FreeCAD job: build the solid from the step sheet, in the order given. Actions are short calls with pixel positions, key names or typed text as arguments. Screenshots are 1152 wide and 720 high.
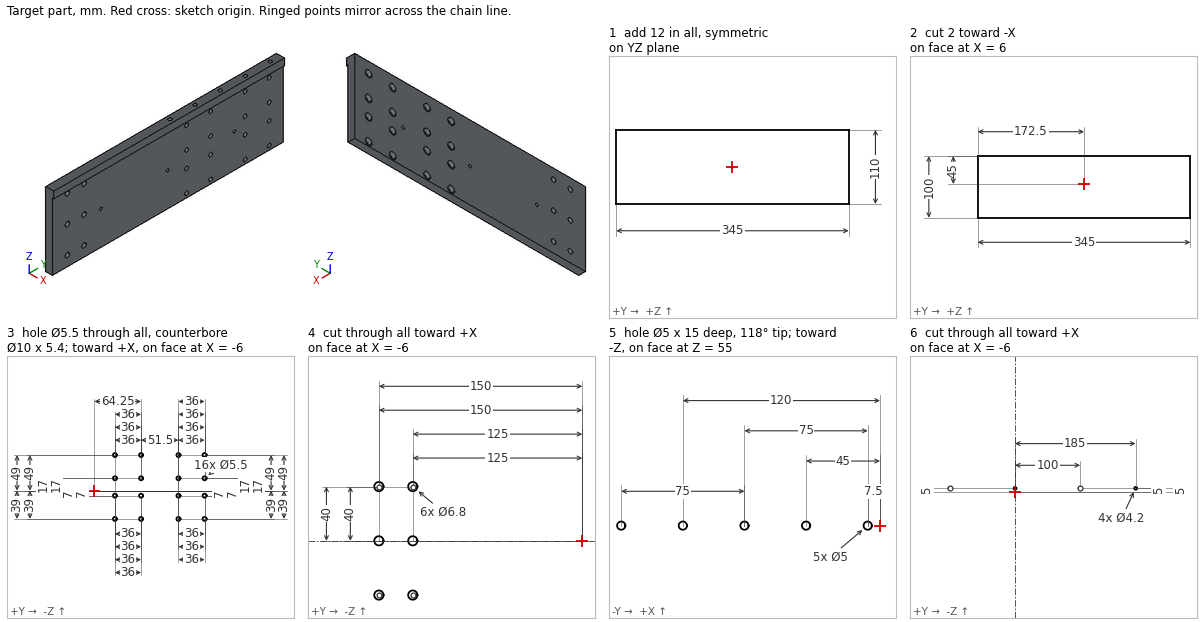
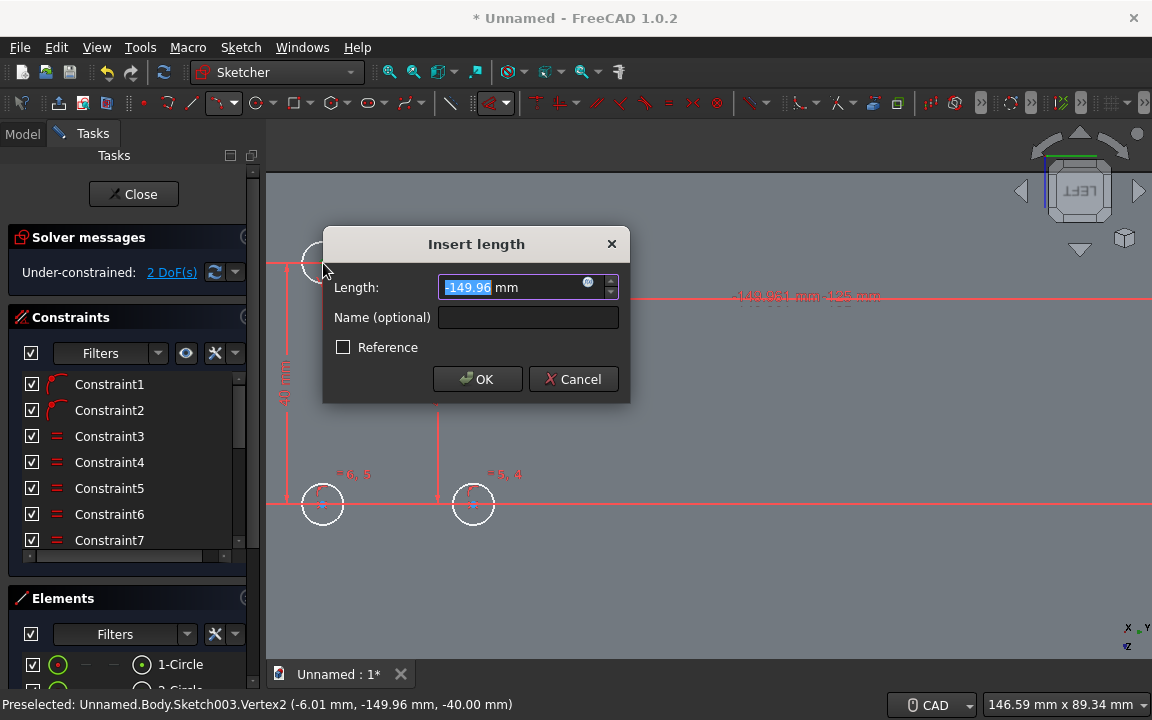
text(-150)
key(Return)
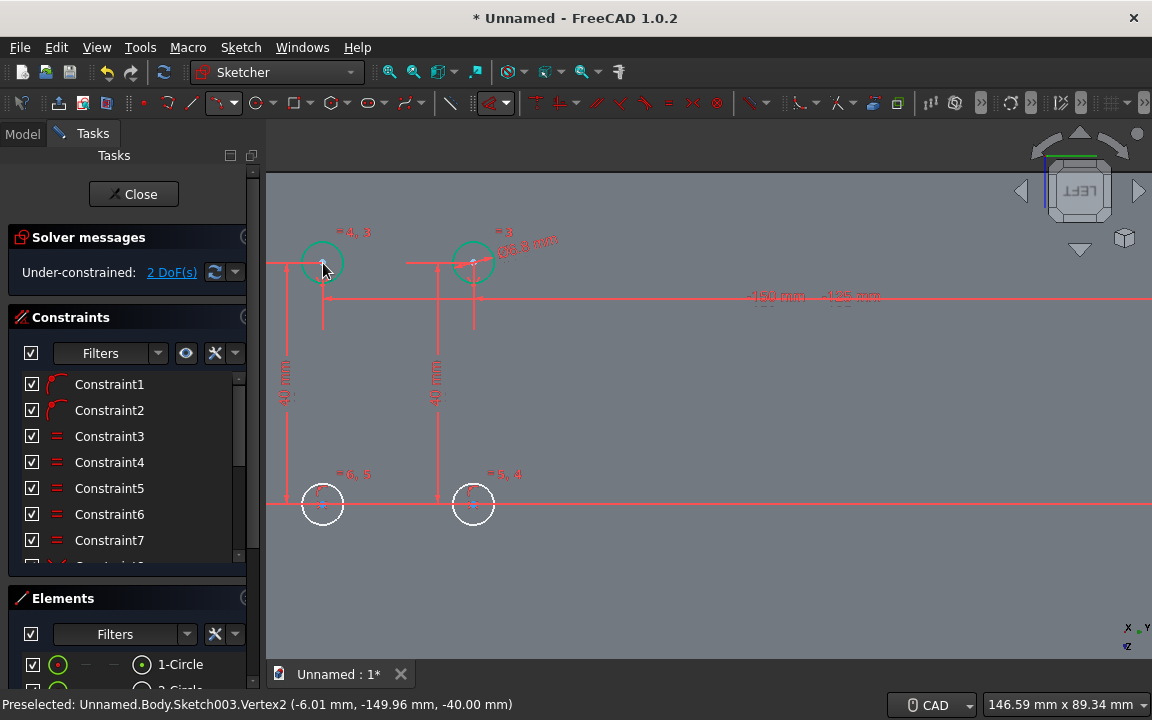
click(473, 504)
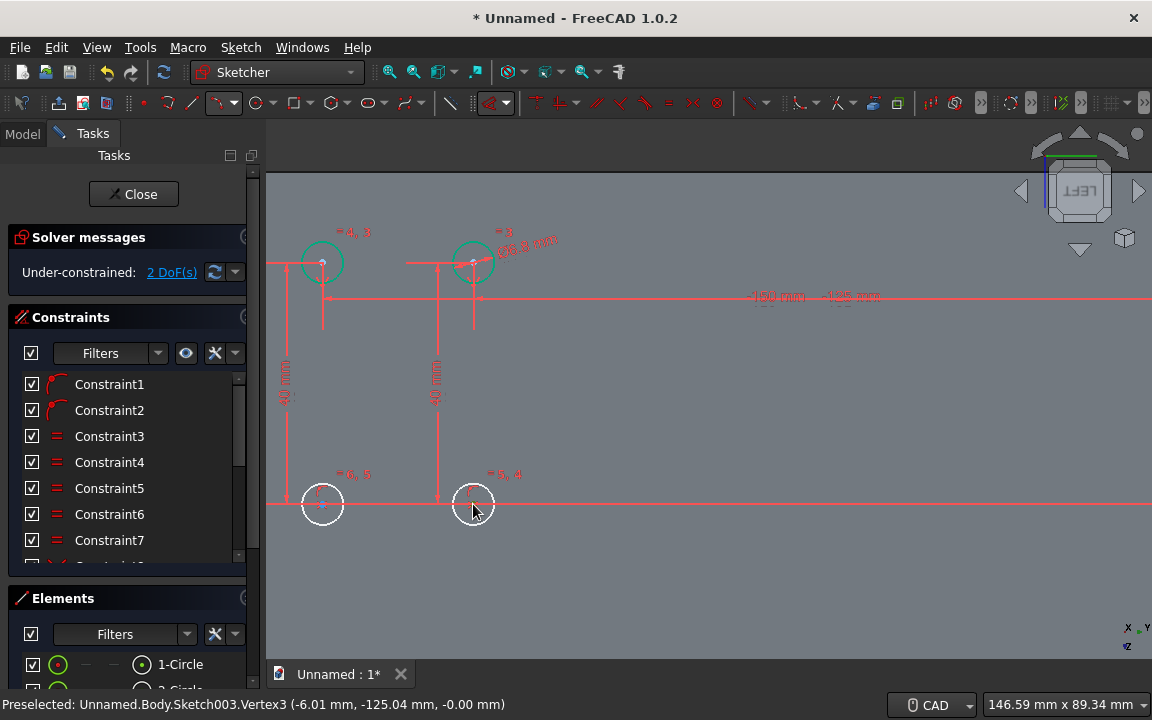
key(l)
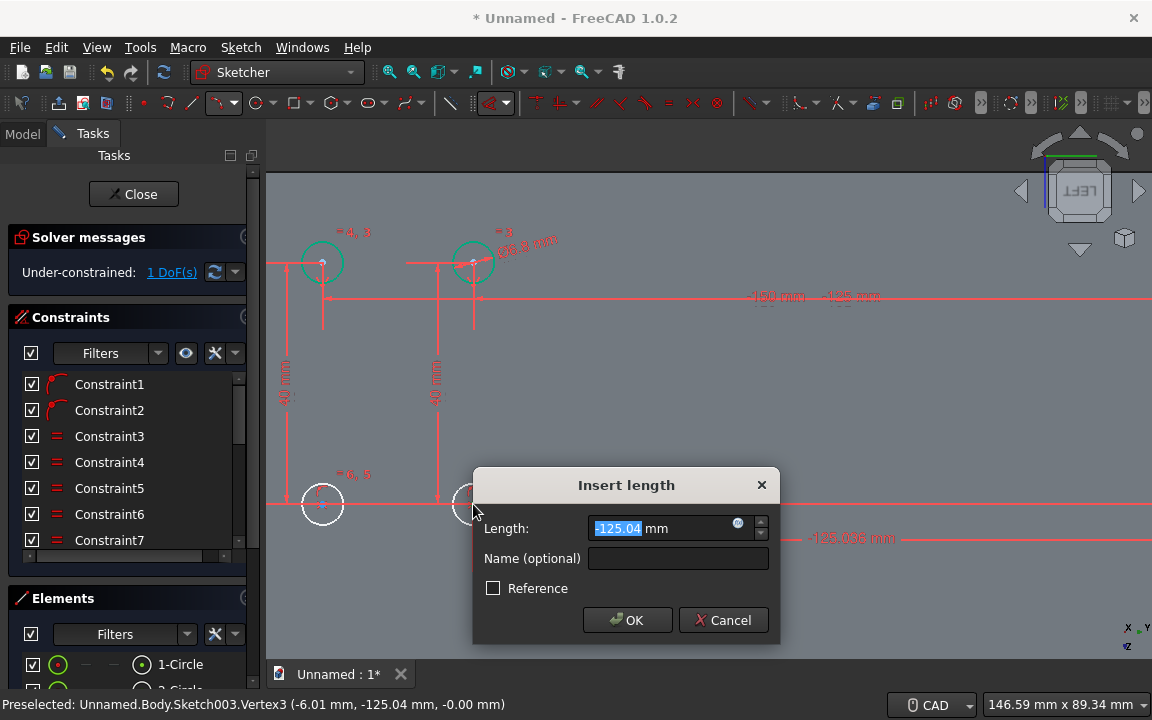
text(-125)
key(Return)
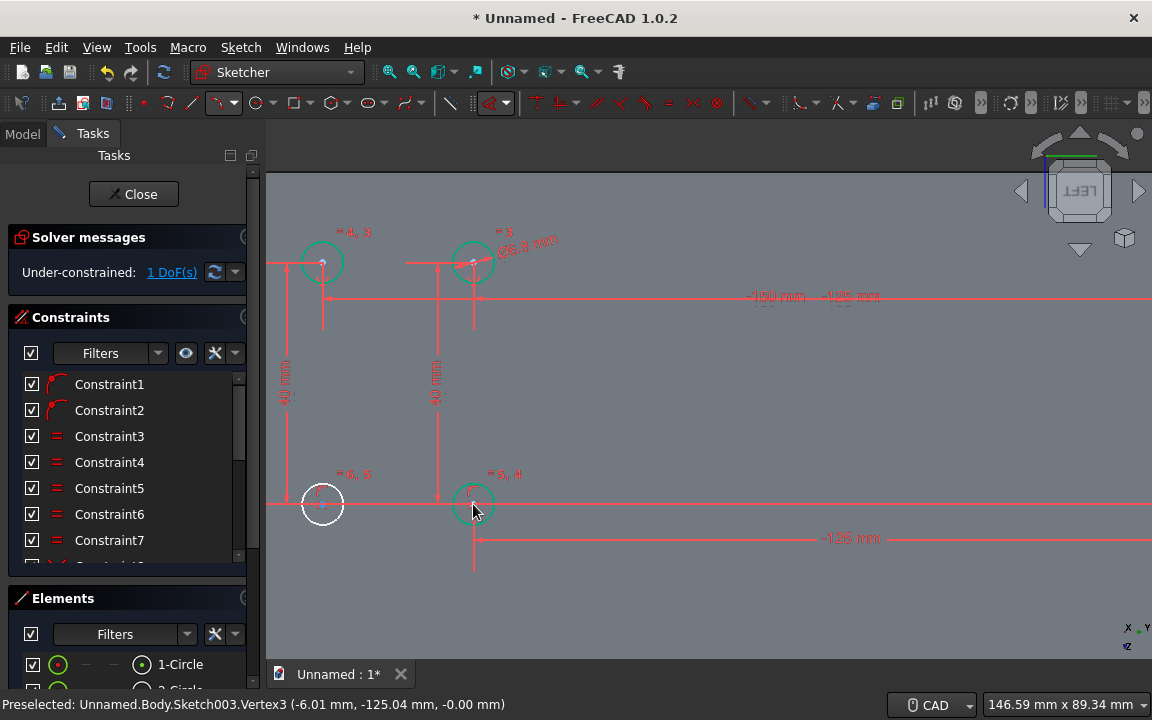
click(323, 504)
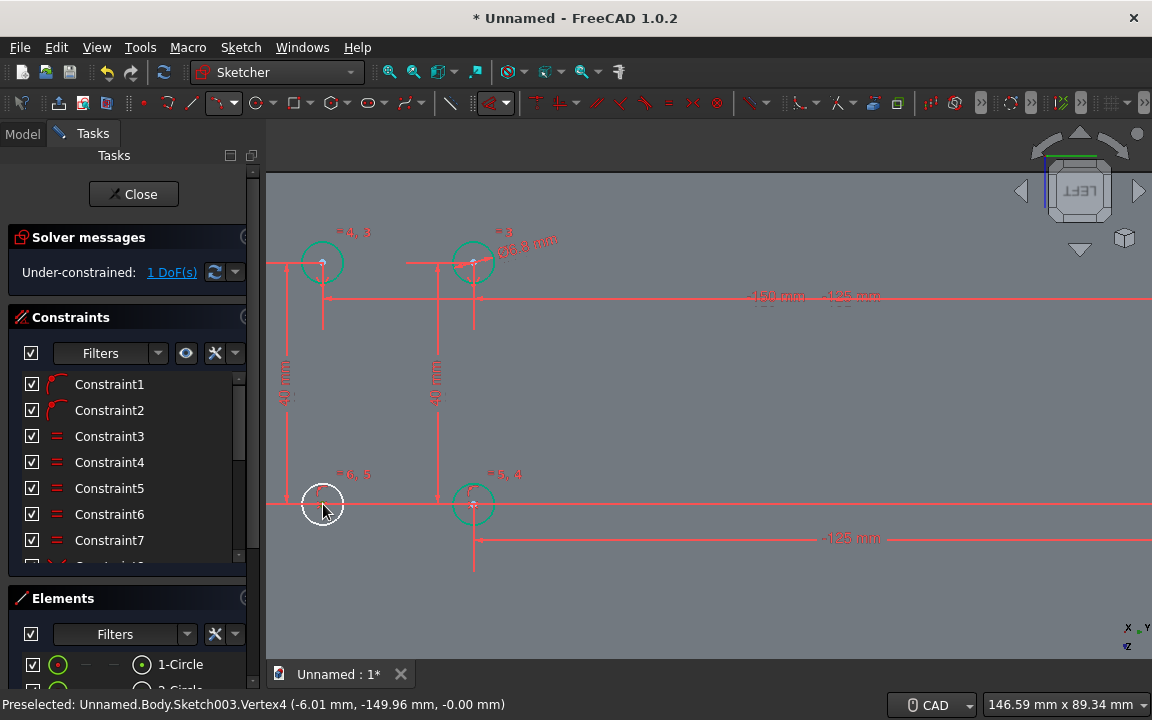
key(l)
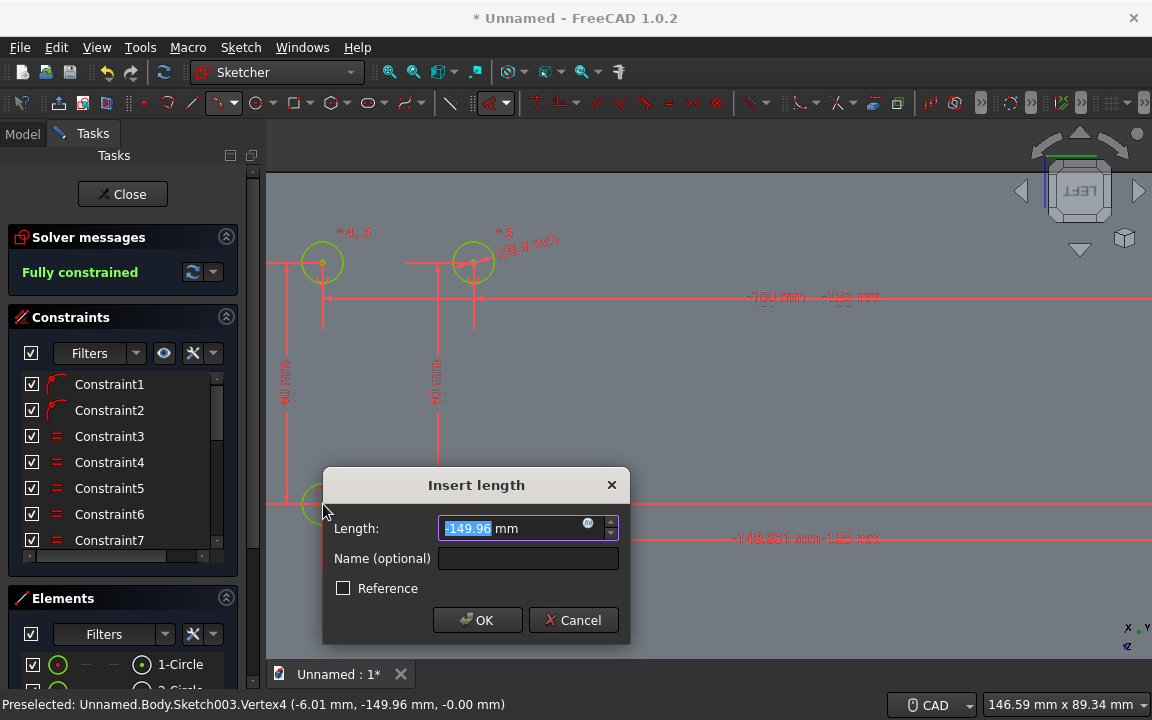
text(-150)
key(Return)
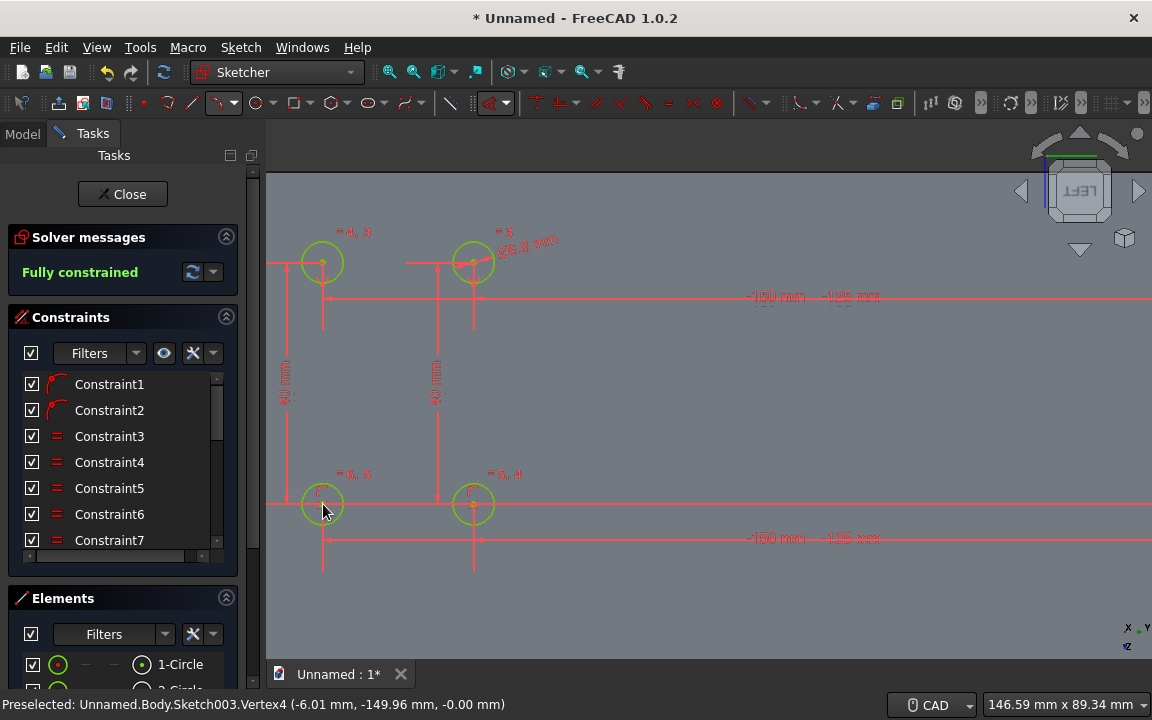
click(123, 194)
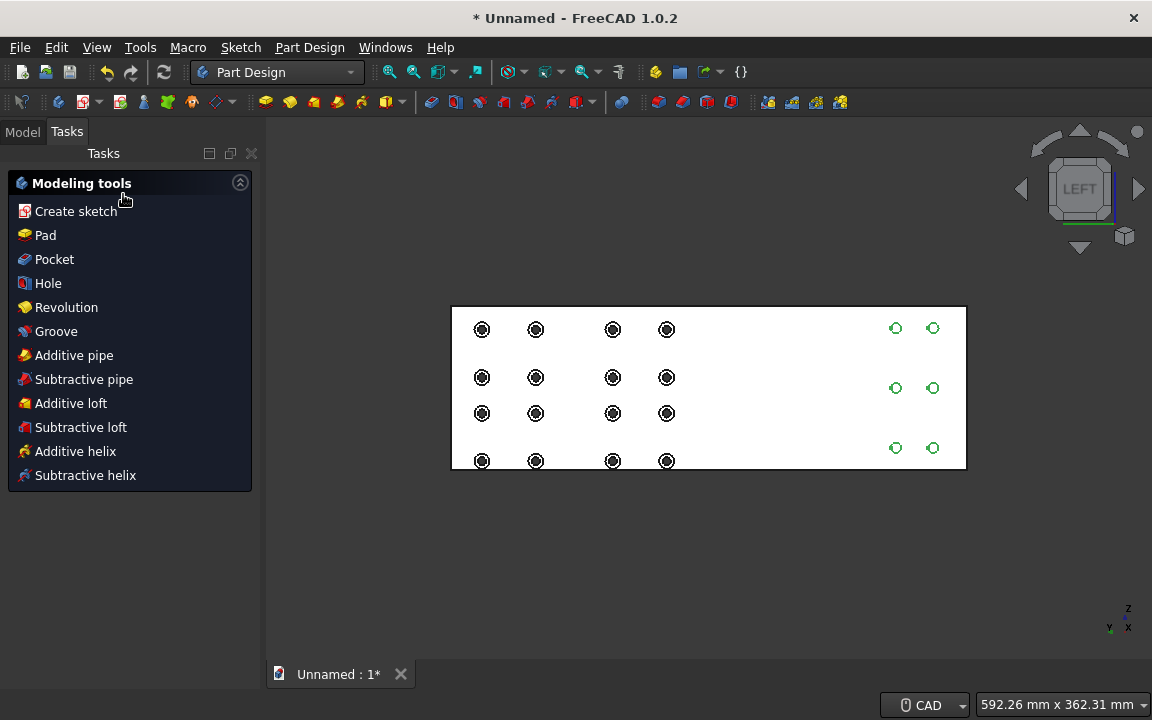
click(432, 102)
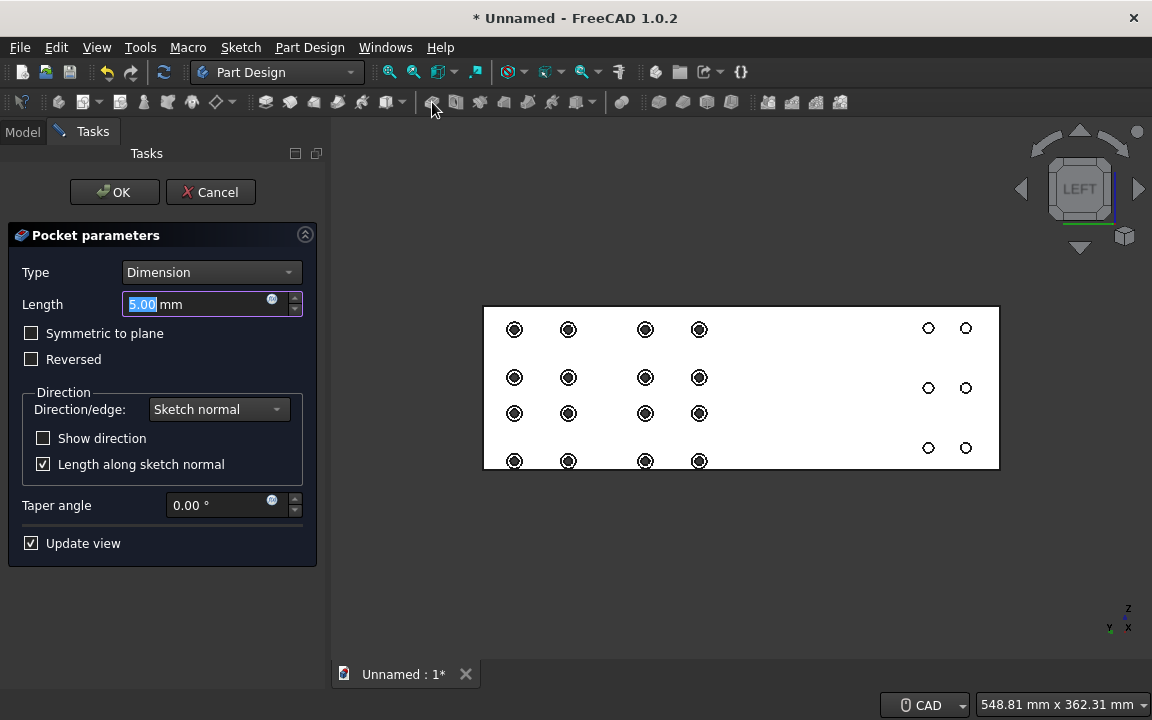
click(212, 272)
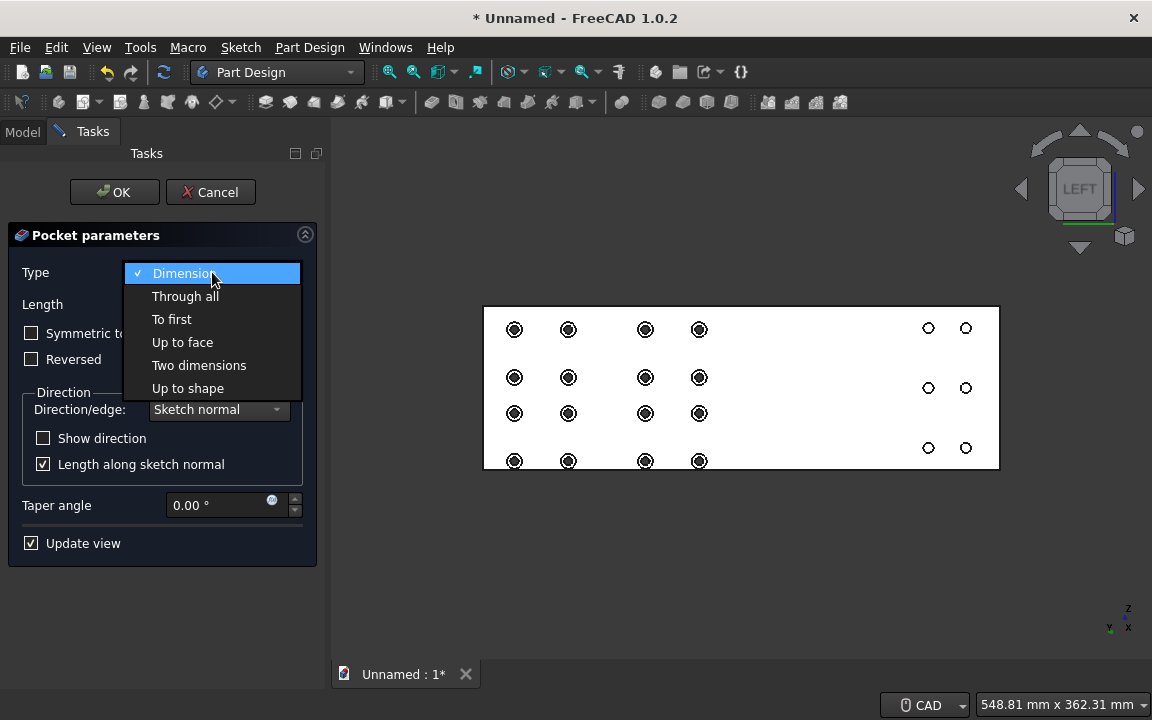
click(212, 296)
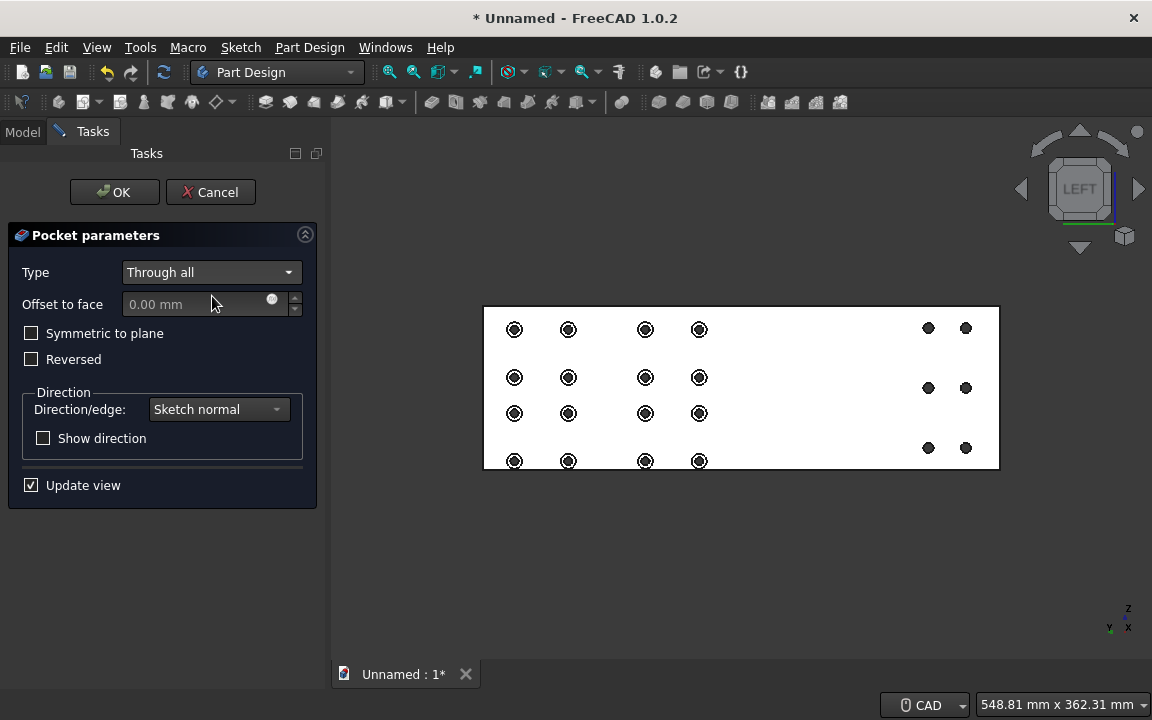
click(115, 192)